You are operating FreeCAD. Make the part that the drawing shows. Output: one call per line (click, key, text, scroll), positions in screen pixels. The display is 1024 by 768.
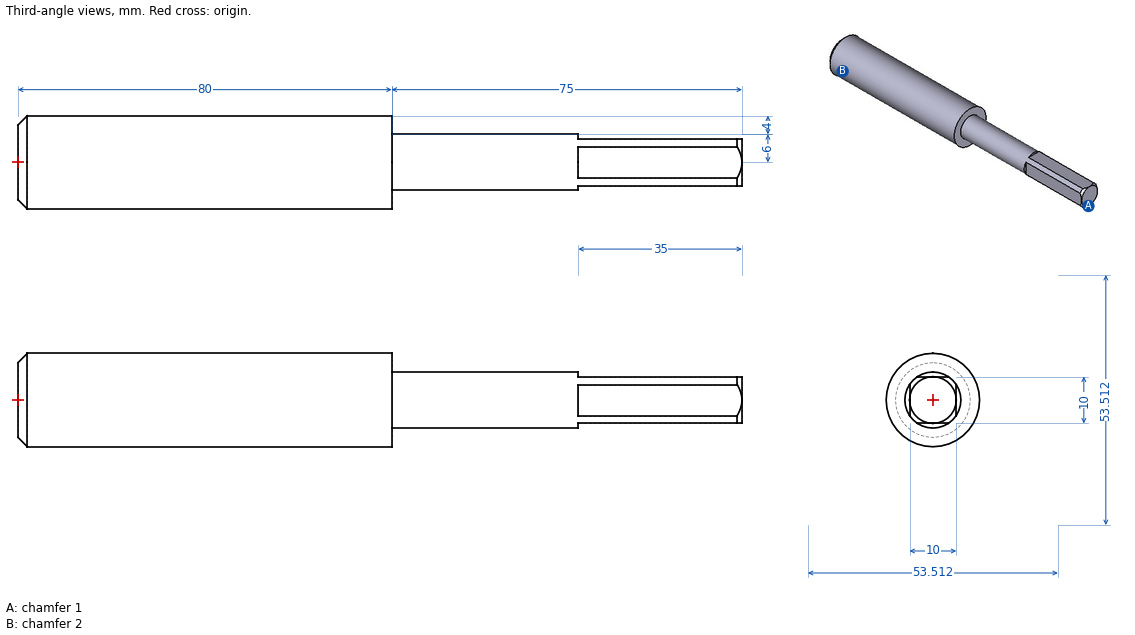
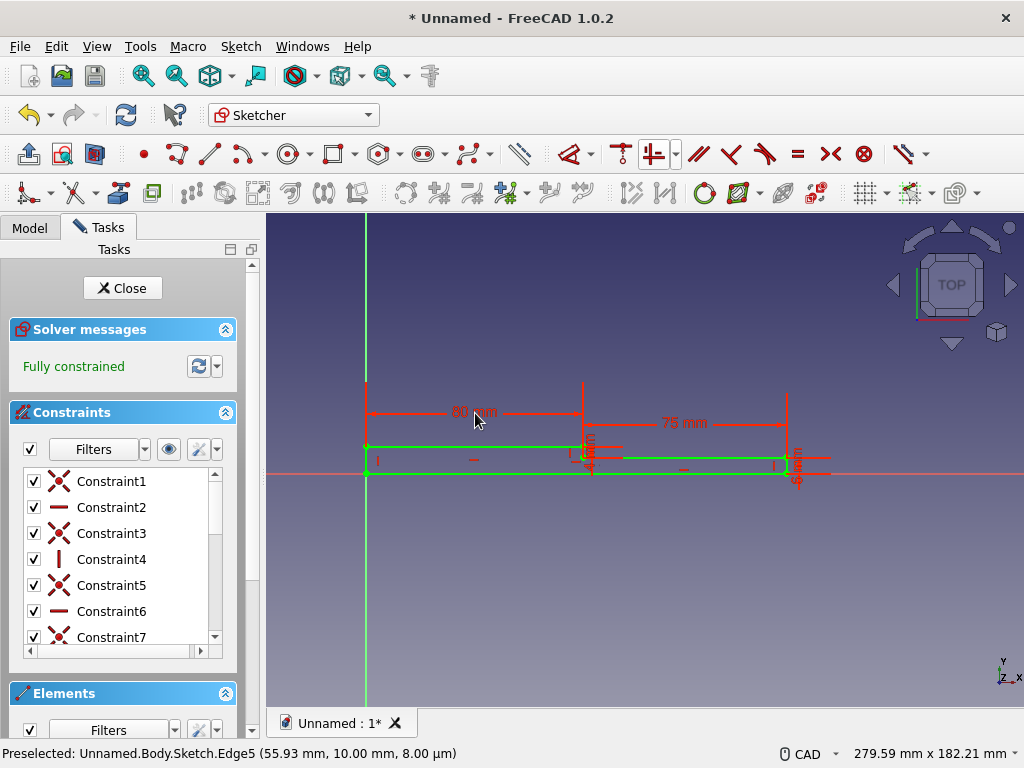
click(123, 288)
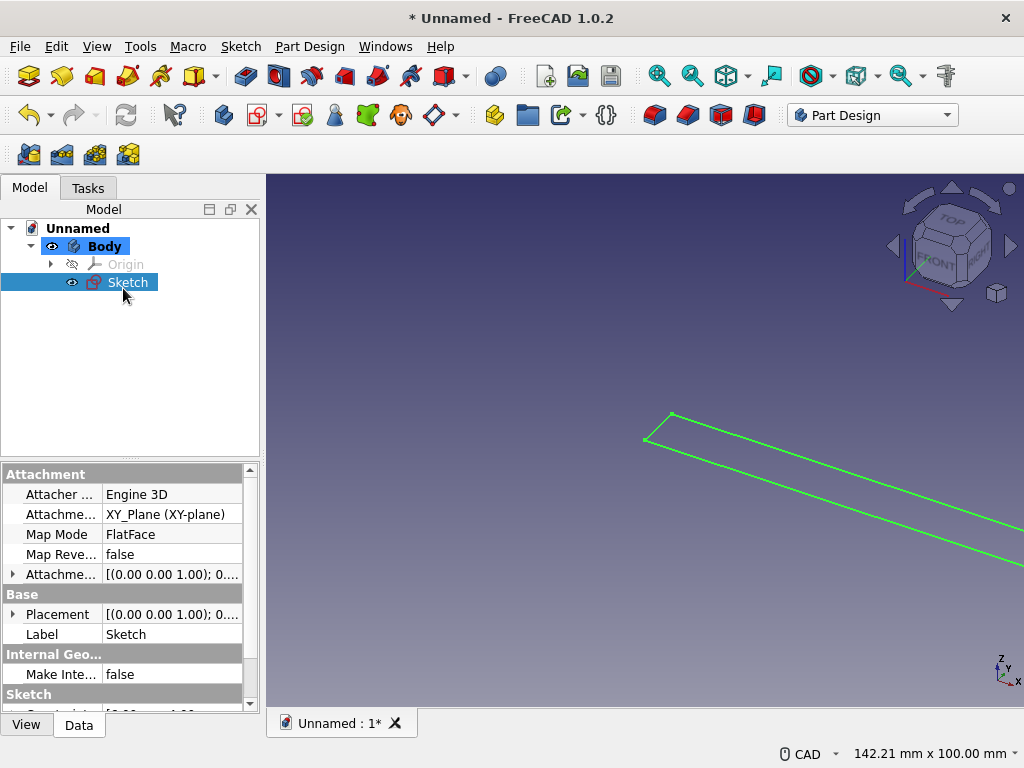
click(62, 76)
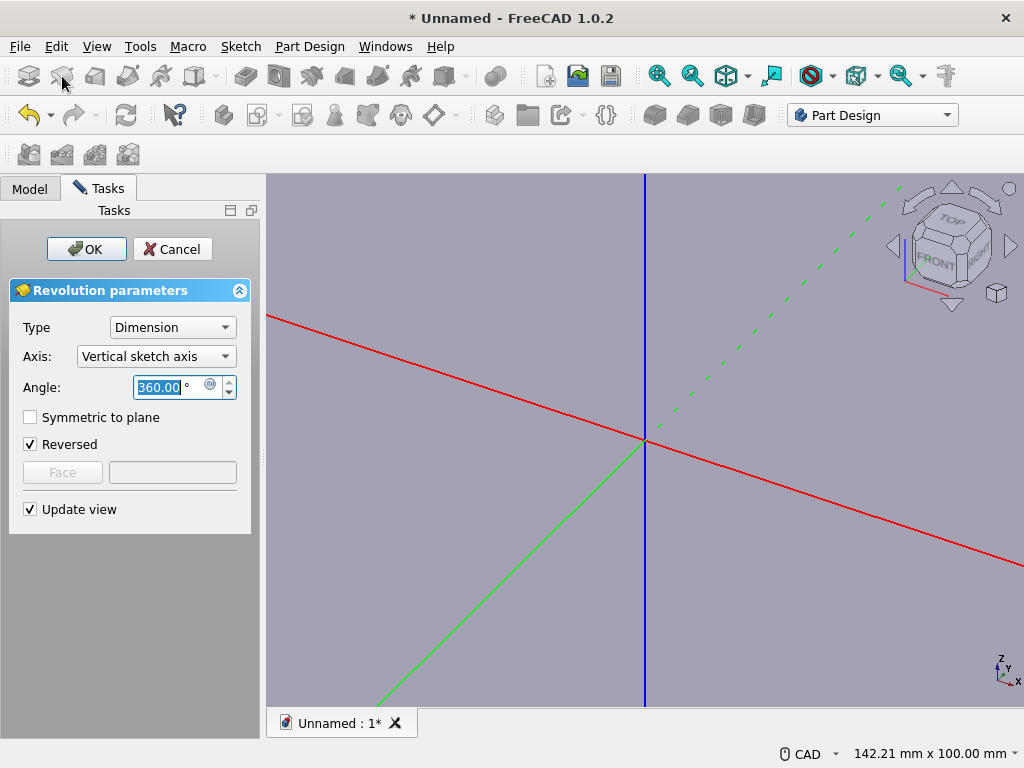
click(157, 356)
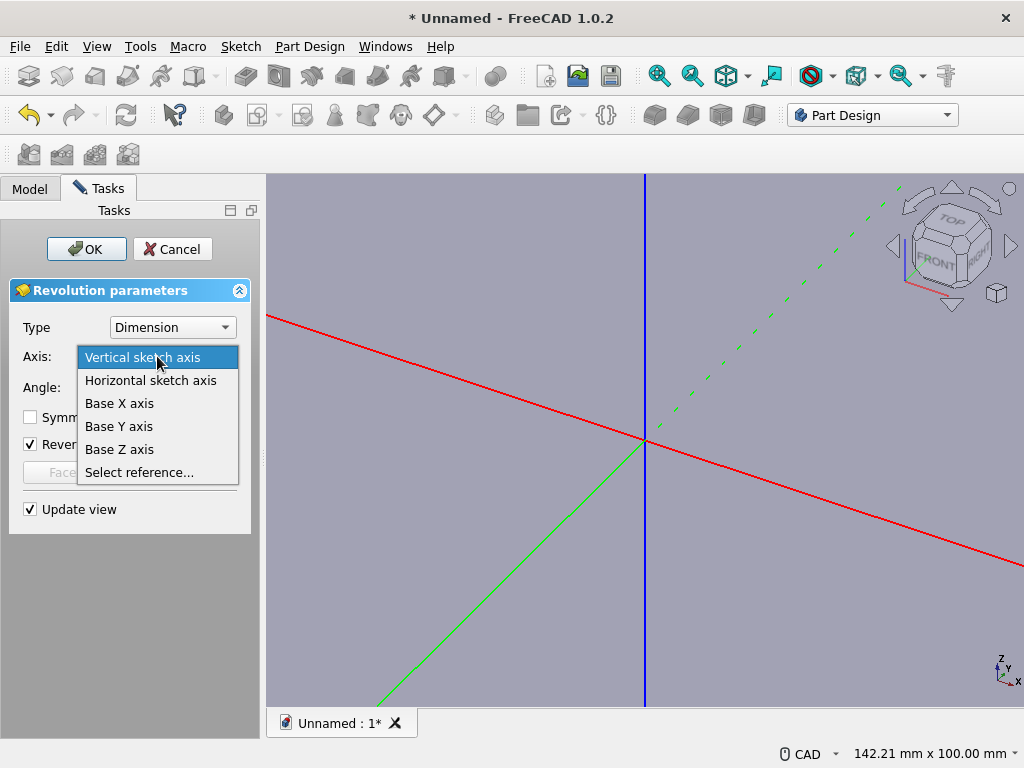
click(156, 380)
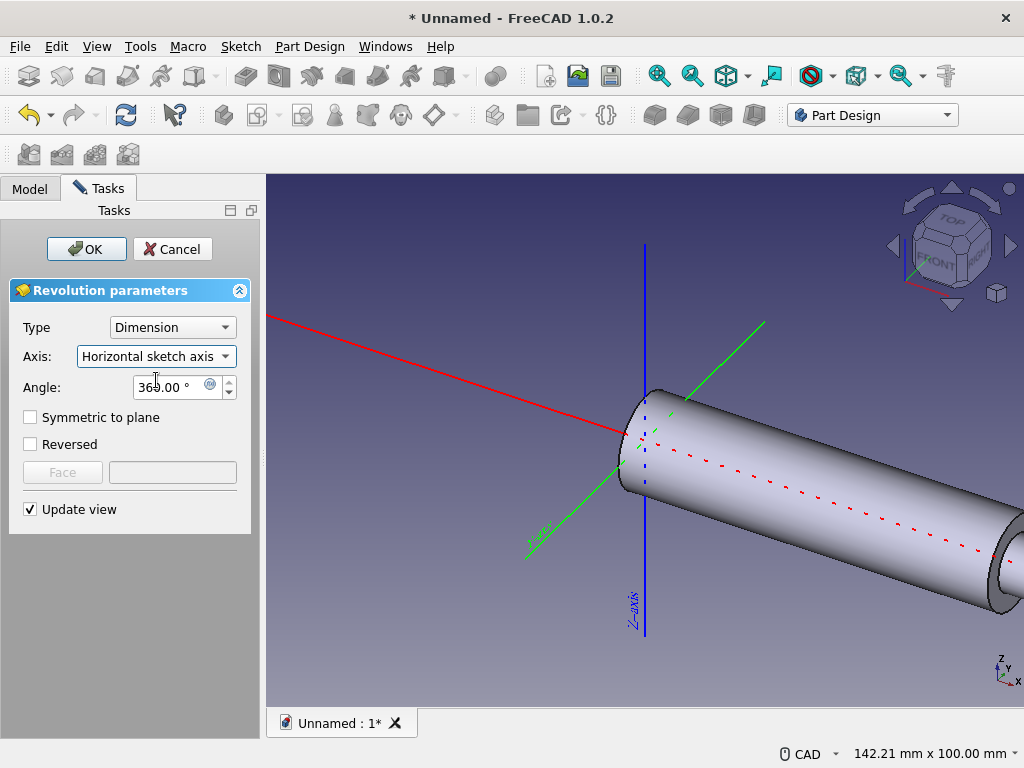
click(87, 249)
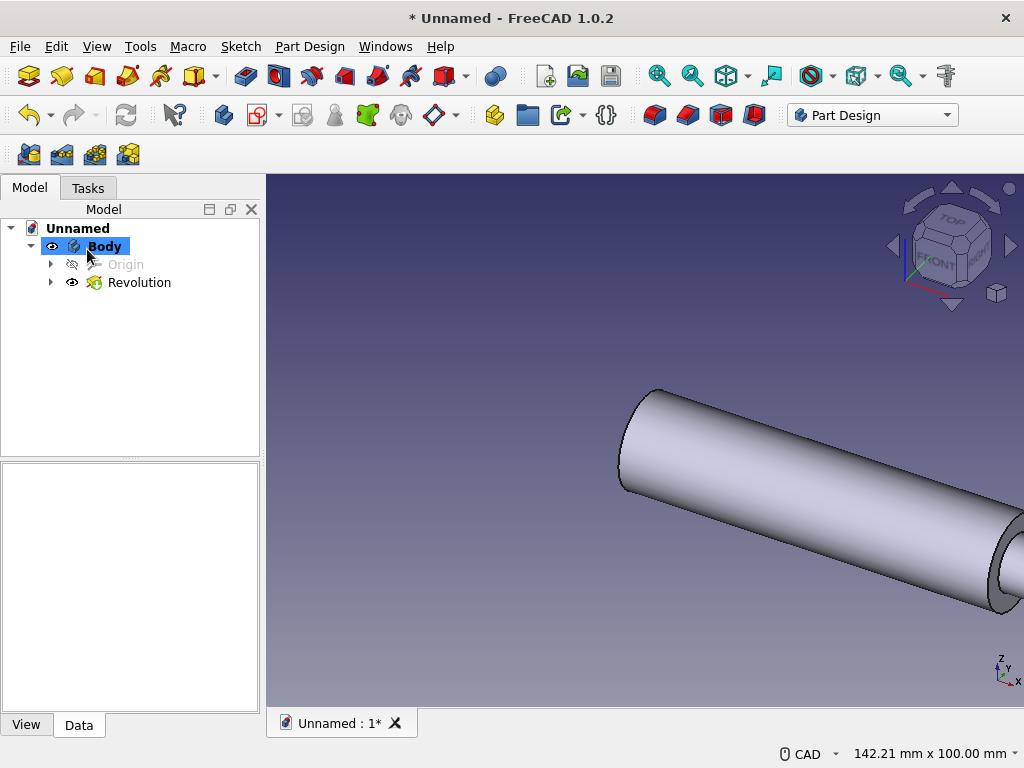
key(v)
key(f)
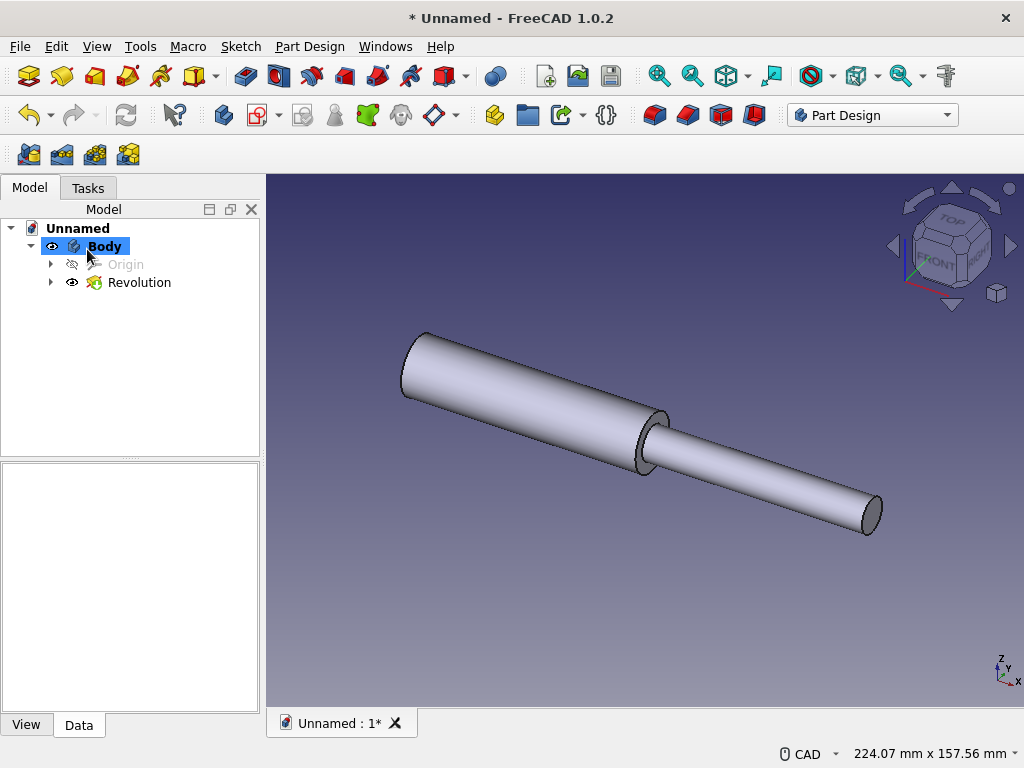
click(862, 525)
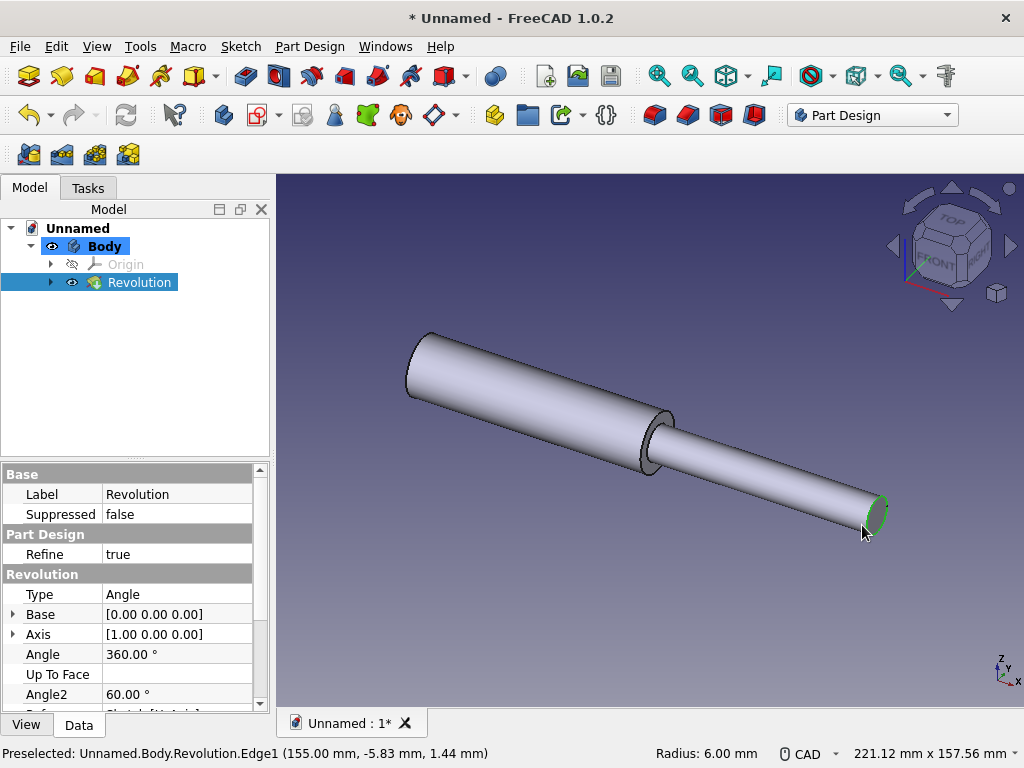
click(688, 116)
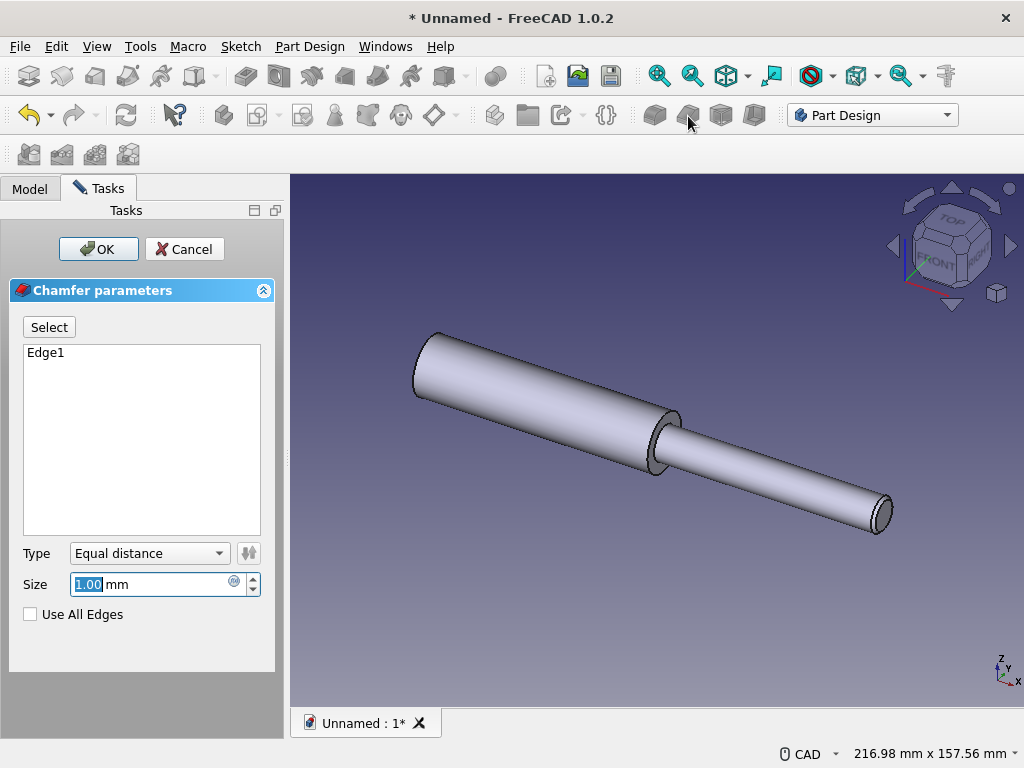
text(1)
key(Tab)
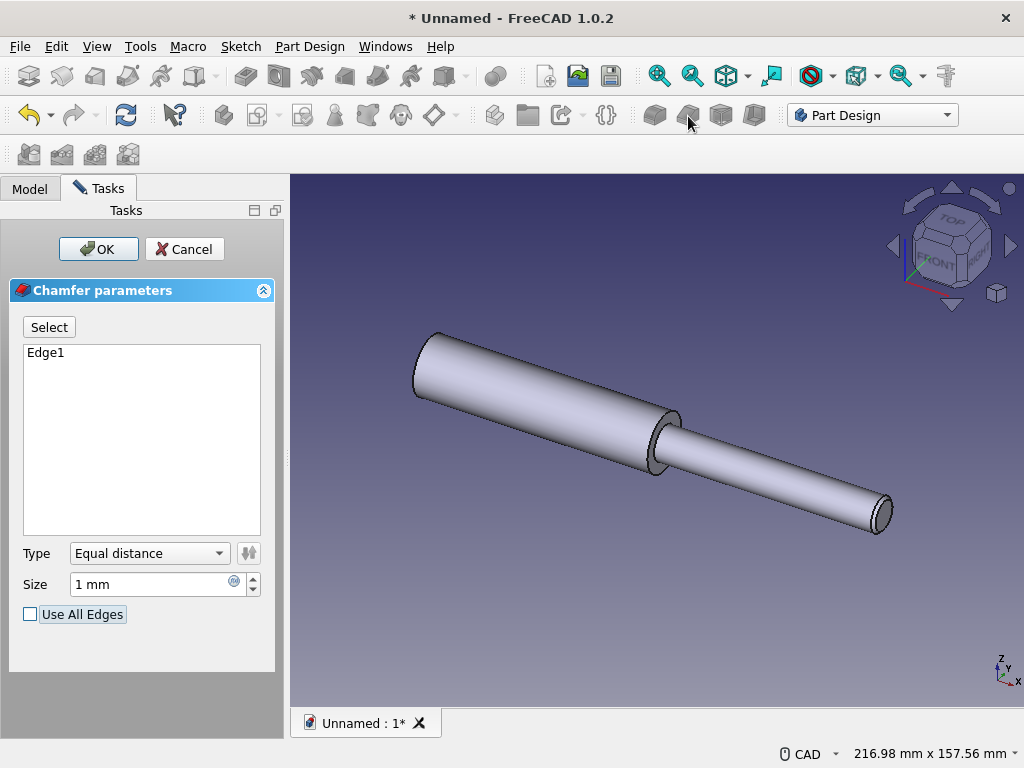
click(99, 249)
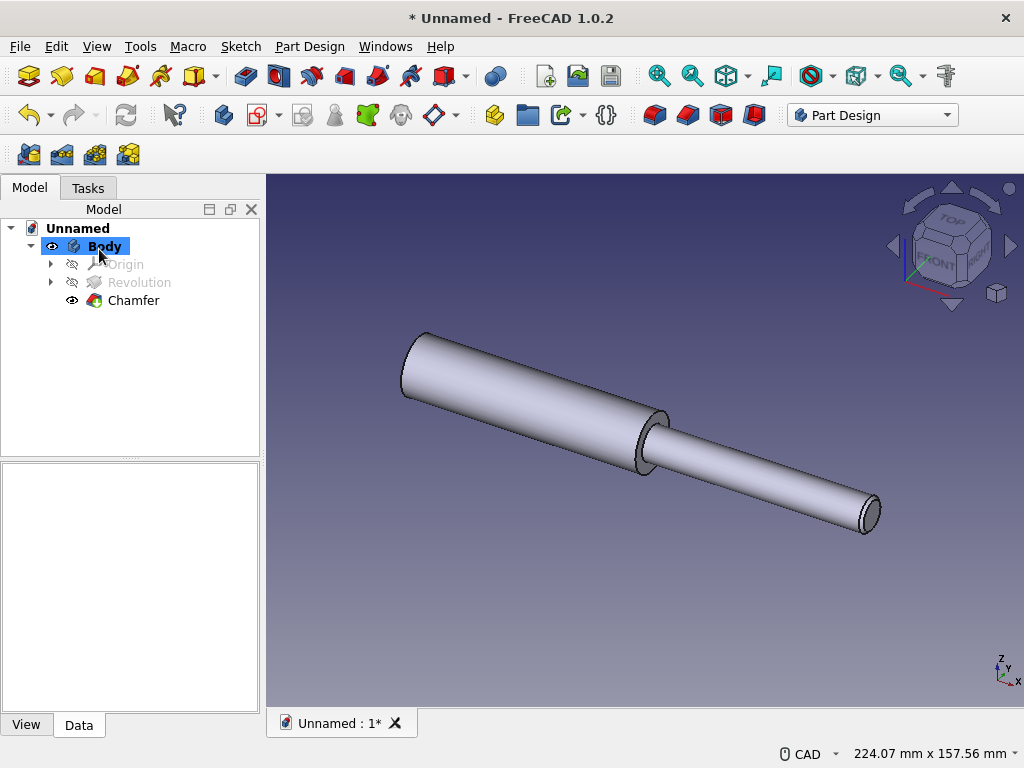
click(404, 394)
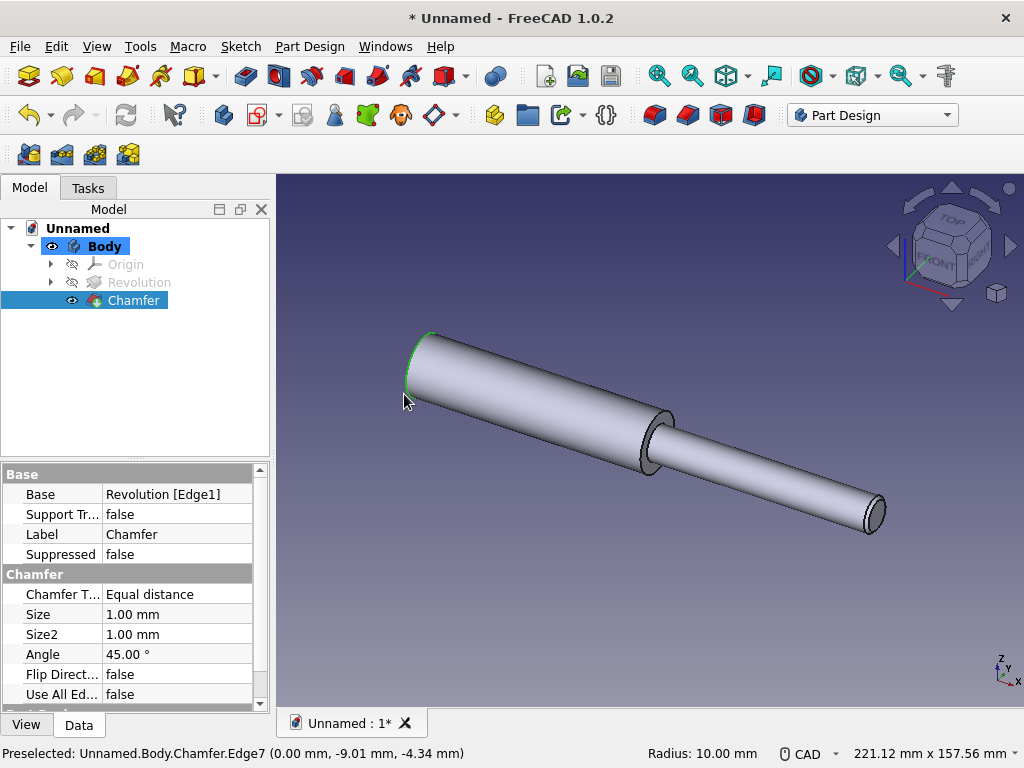
click(688, 116)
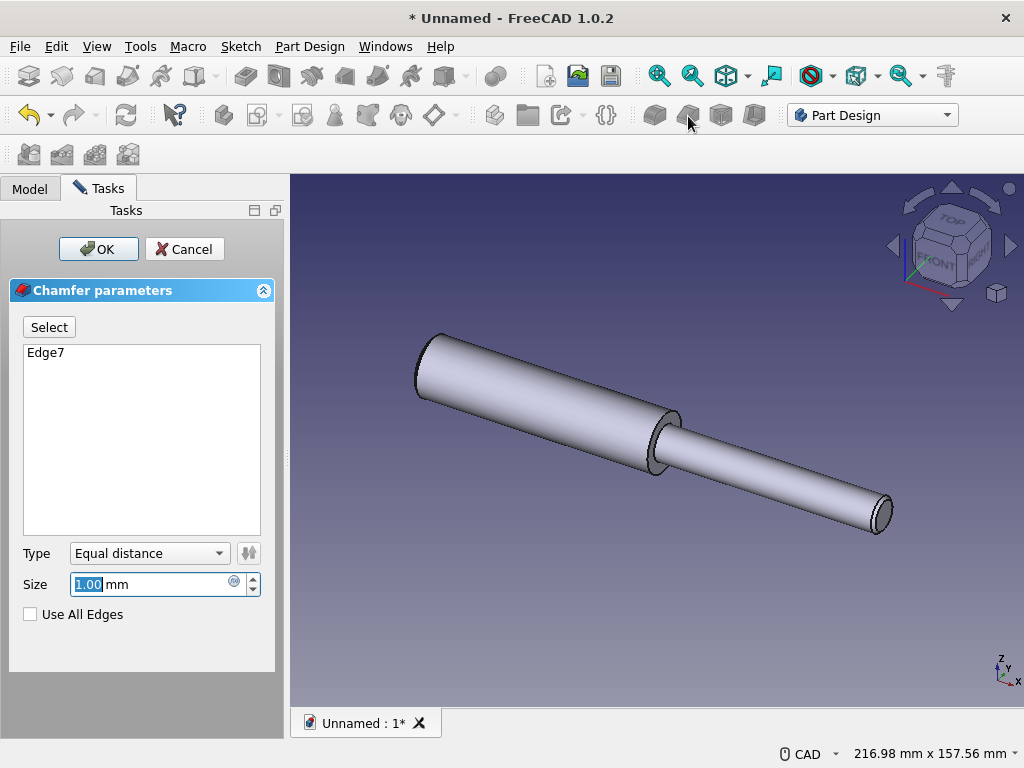
text(2)
key(Tab)